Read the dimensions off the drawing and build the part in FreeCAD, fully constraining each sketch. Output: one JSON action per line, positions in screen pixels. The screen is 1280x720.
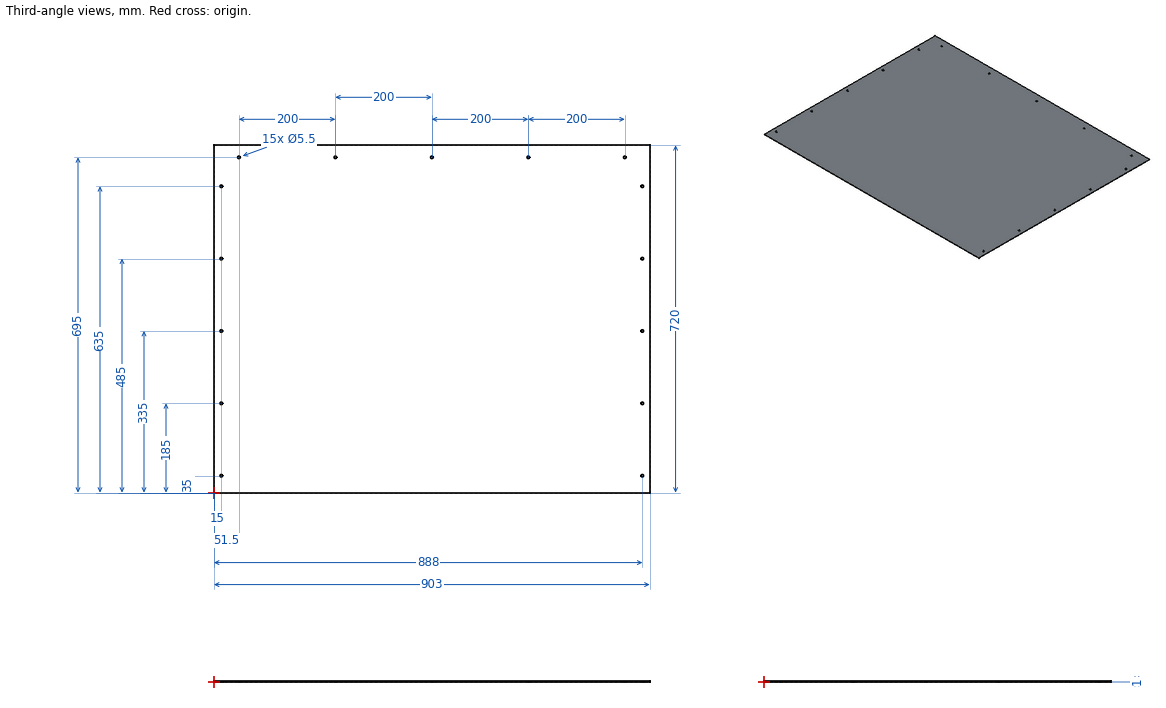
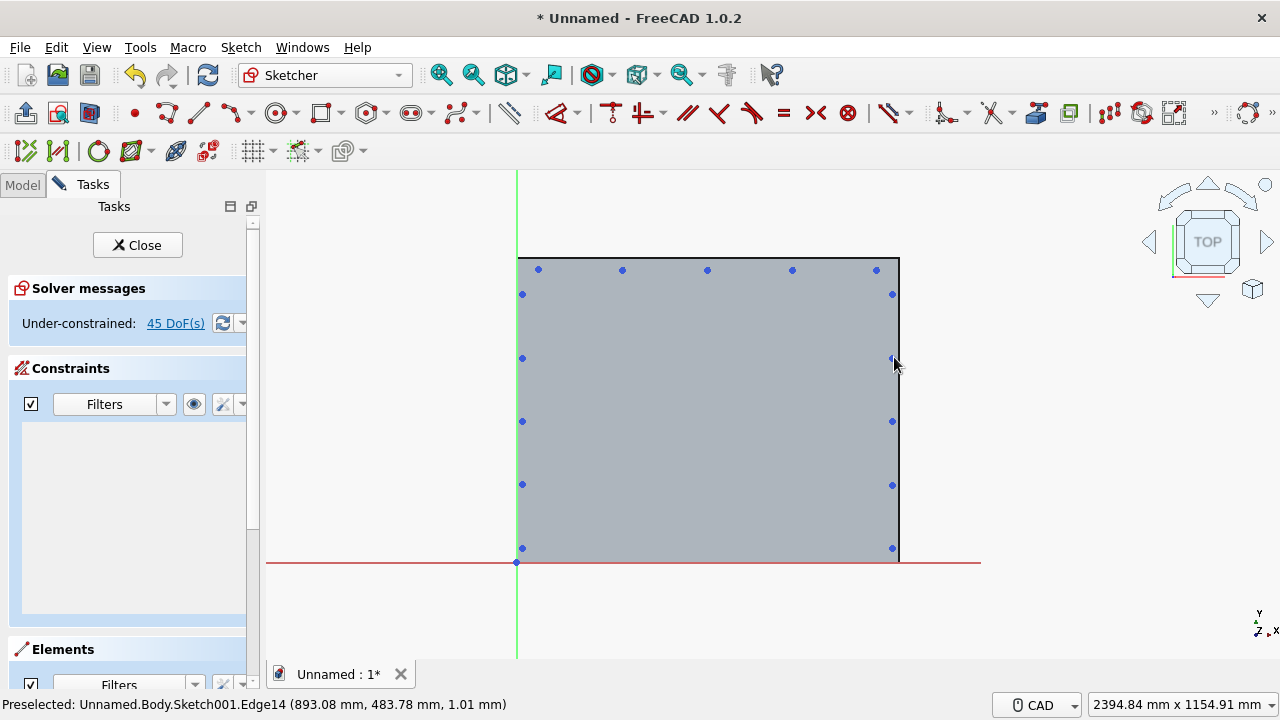
{"action": "scroll", "coordinate": [894, 294], "scroll_direction": "up", "scroll_amount": 11}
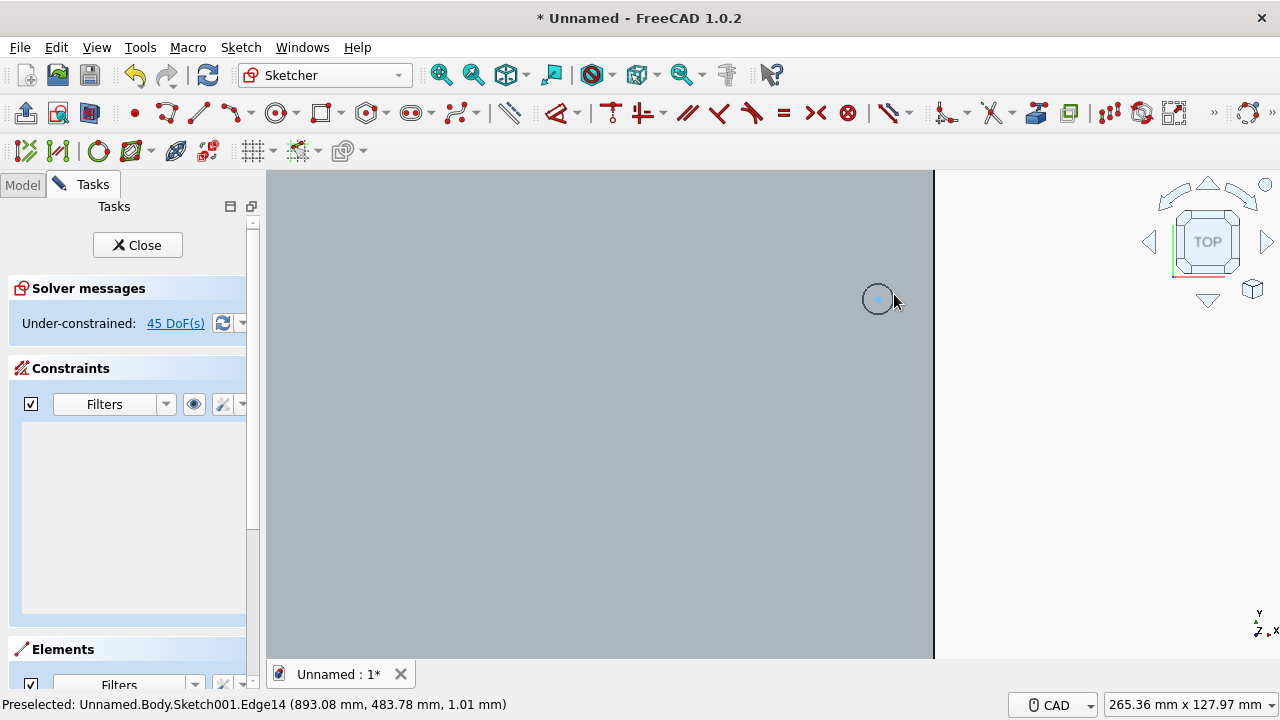
{"action": "left_click", "coordinate": [889, 288]}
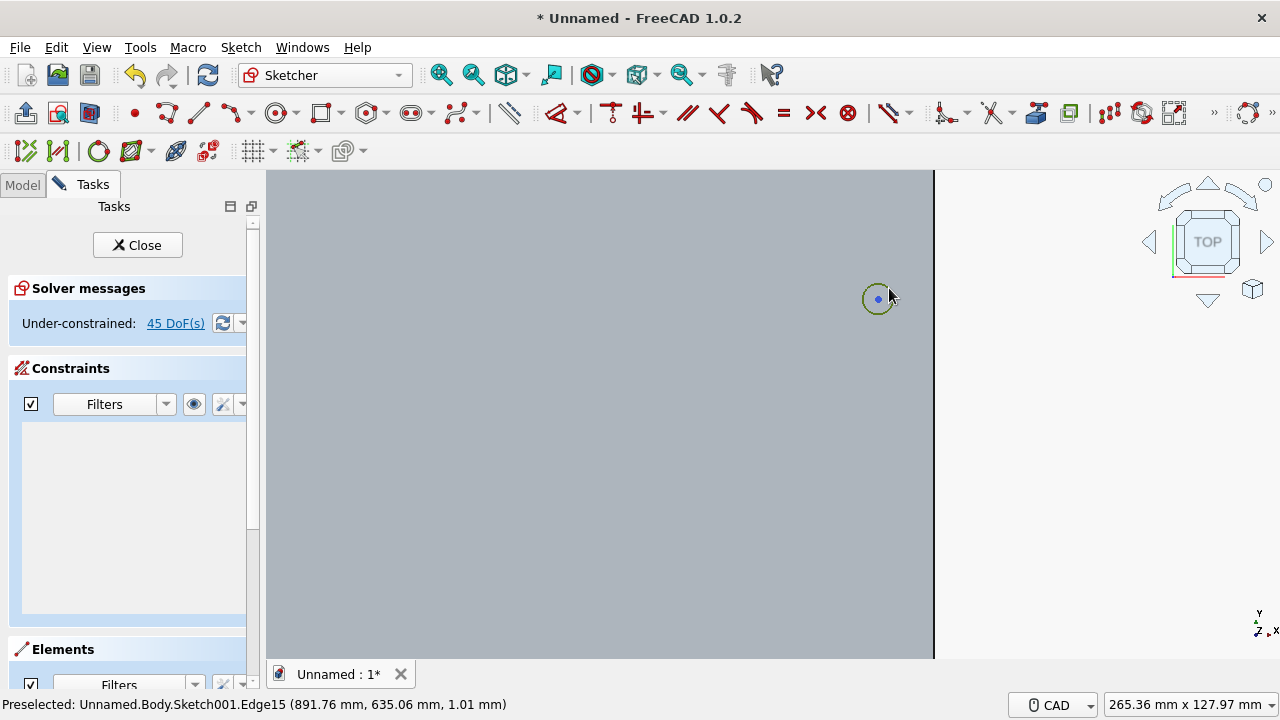
{"action": "left_click", "coordinate": [784, 114]}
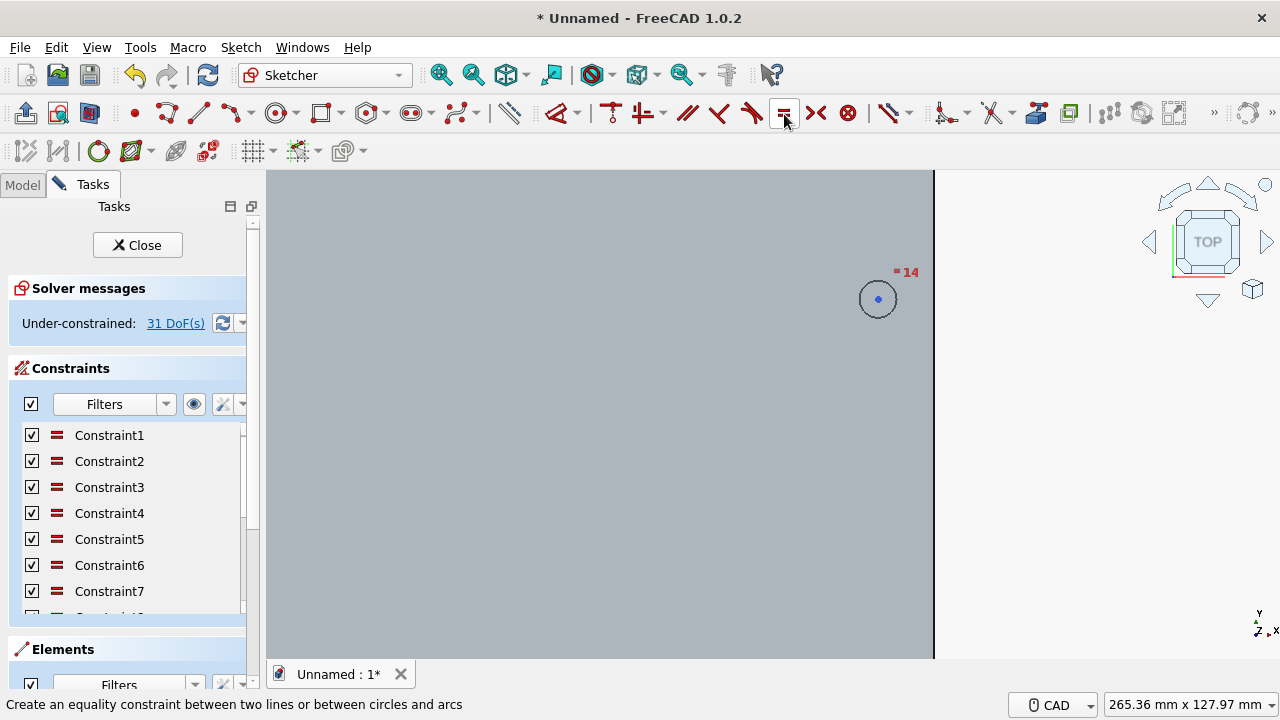
{"action": "key", "text": "d"}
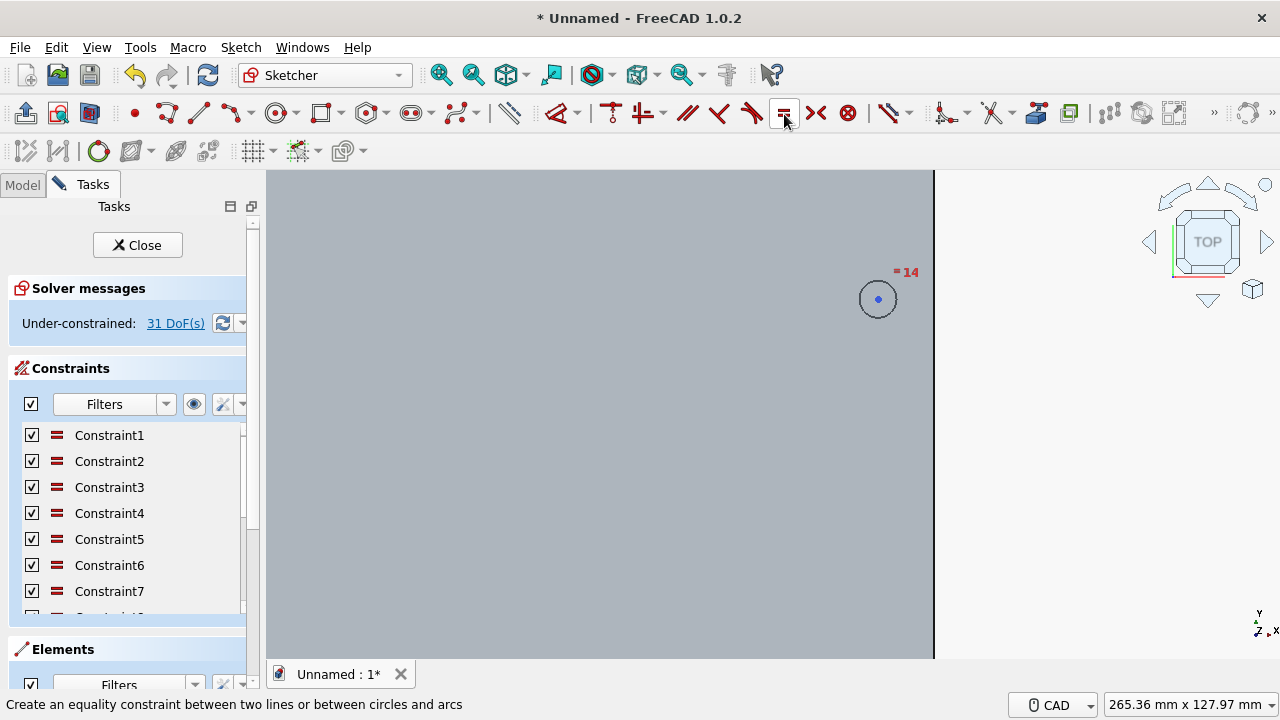
{"action": "scroll", "coordinate": [894, 294], "scroll_direction": "down", "scroll_amount": 11}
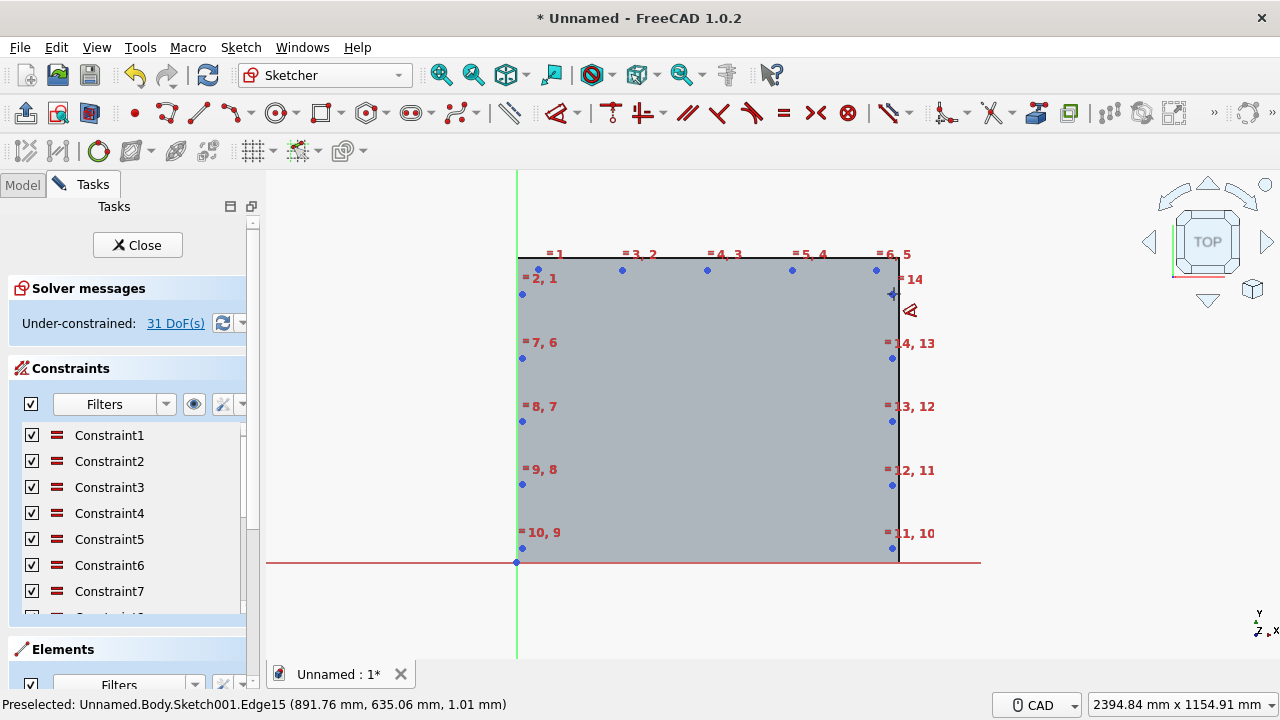
{"action": "scroll", "coordinate": [540, 268], "scroll_direction": "up", "scroll_amount": 15}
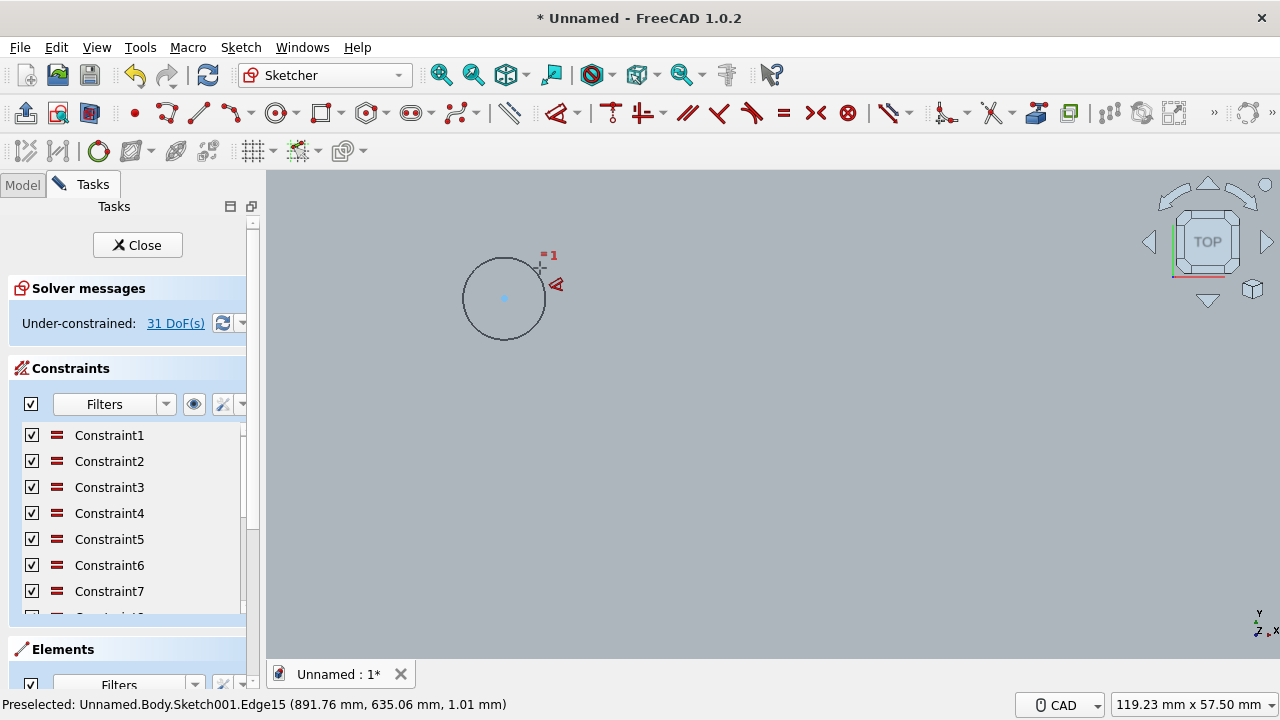
{"action": "left_click", "coordinate": [533, 269]}
{"action": "left_click", "coordinate": [555, 246]}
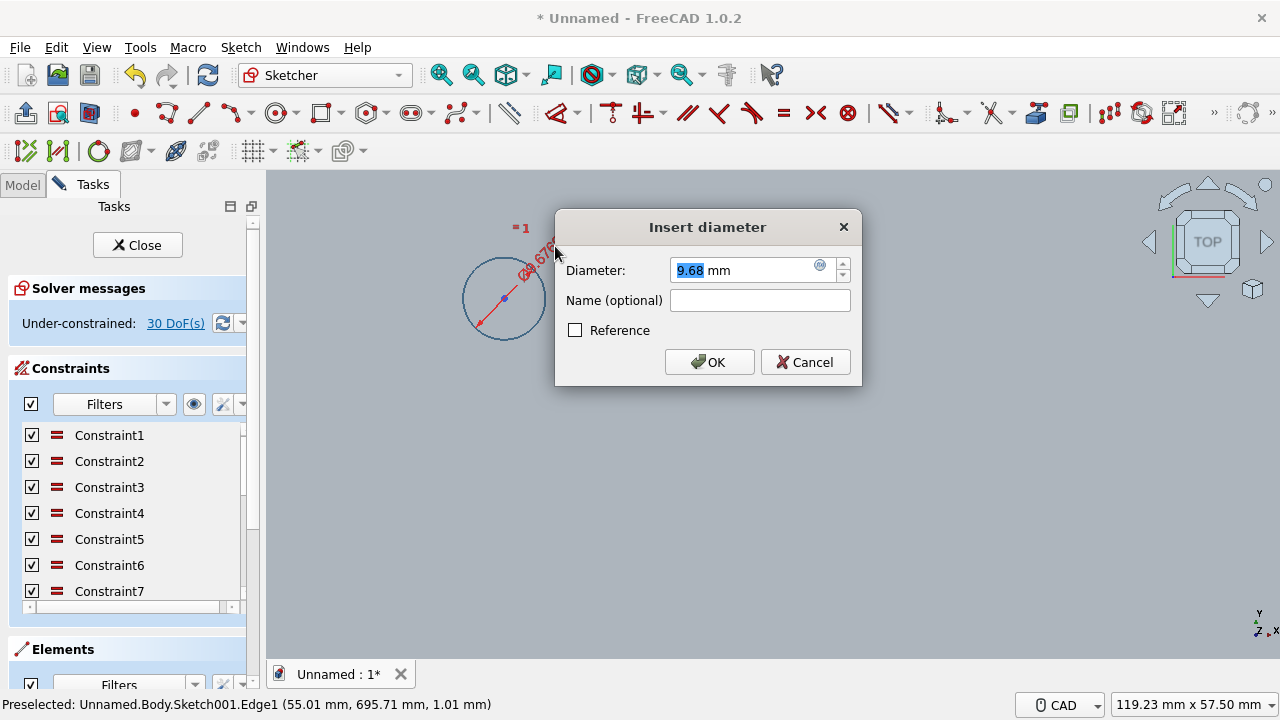
{"action": "type", "text": "5.5"}
{"action": "key", "text": "Return"}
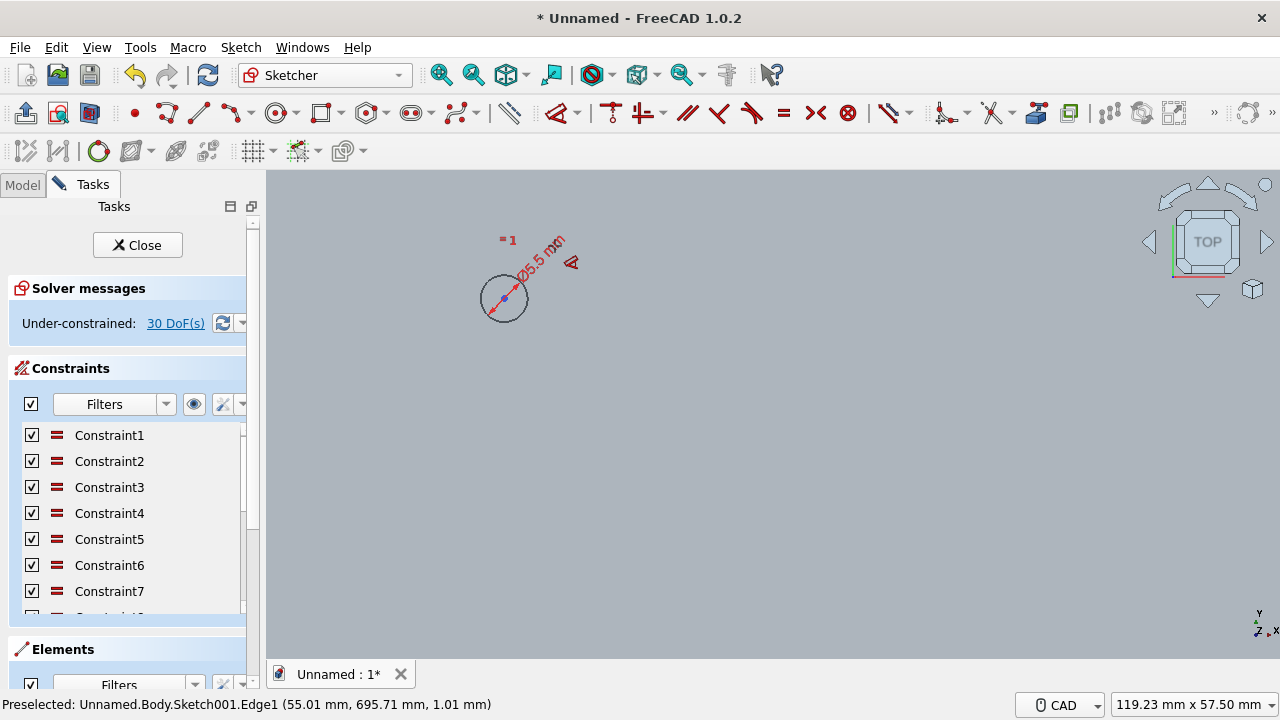
{"action": "scroll", "coordinate": [539, 268], "scroll_direction": "down", "scroll_amount": 15}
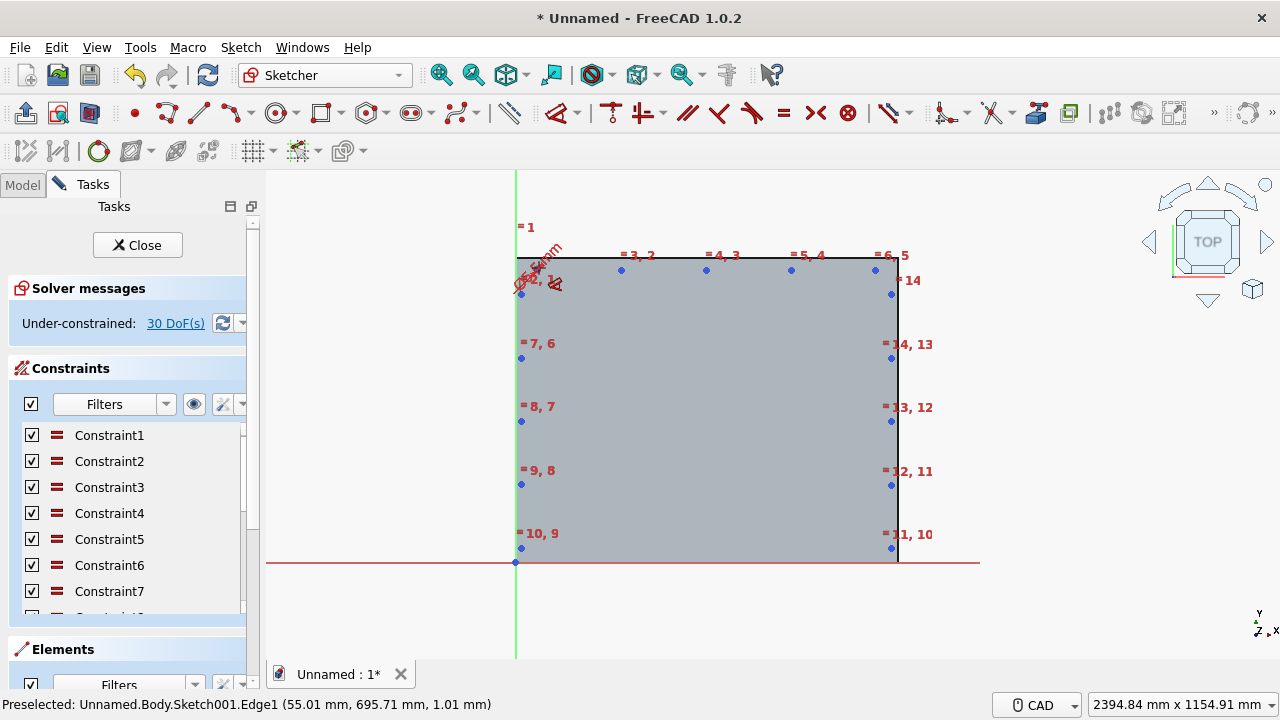
{"action": "scroll", "coordinate": [522, 294], "scroll_direction": "up", "scroll_amount": 10}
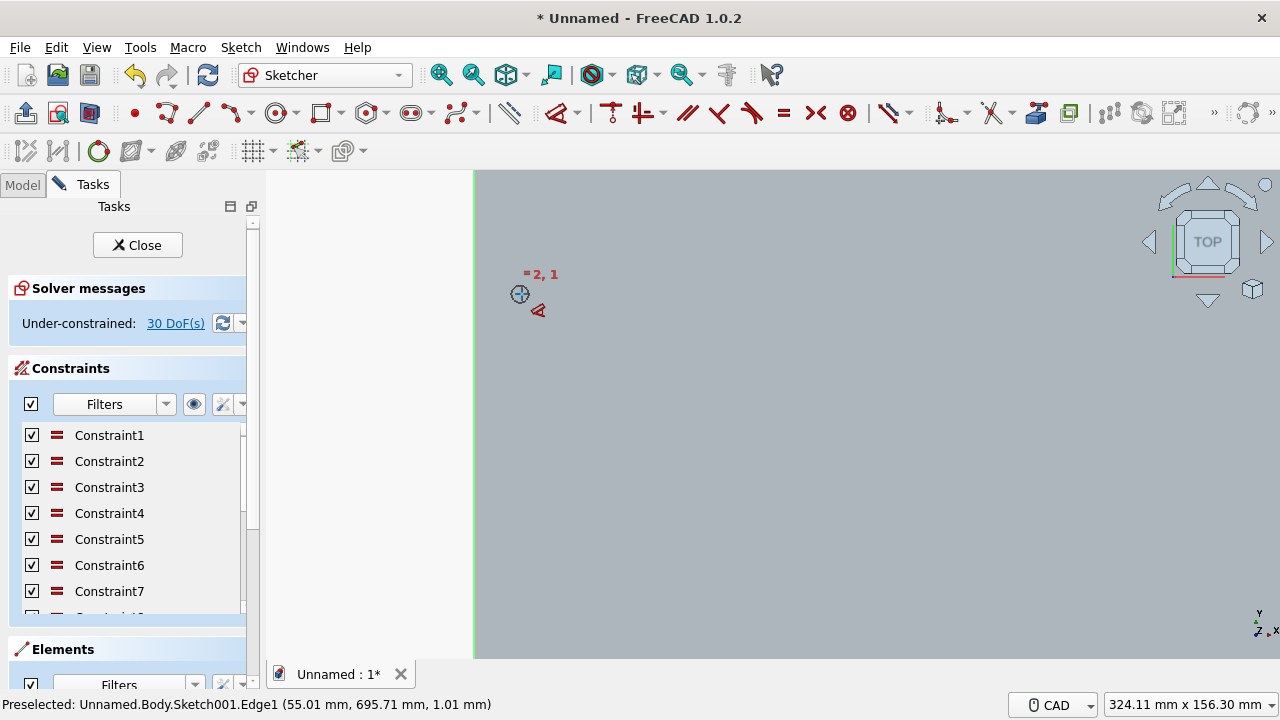
{"action": "left_click", "coordinate": [520, 294]}
{"action": "left_click", "coordinate": [497, 260]}